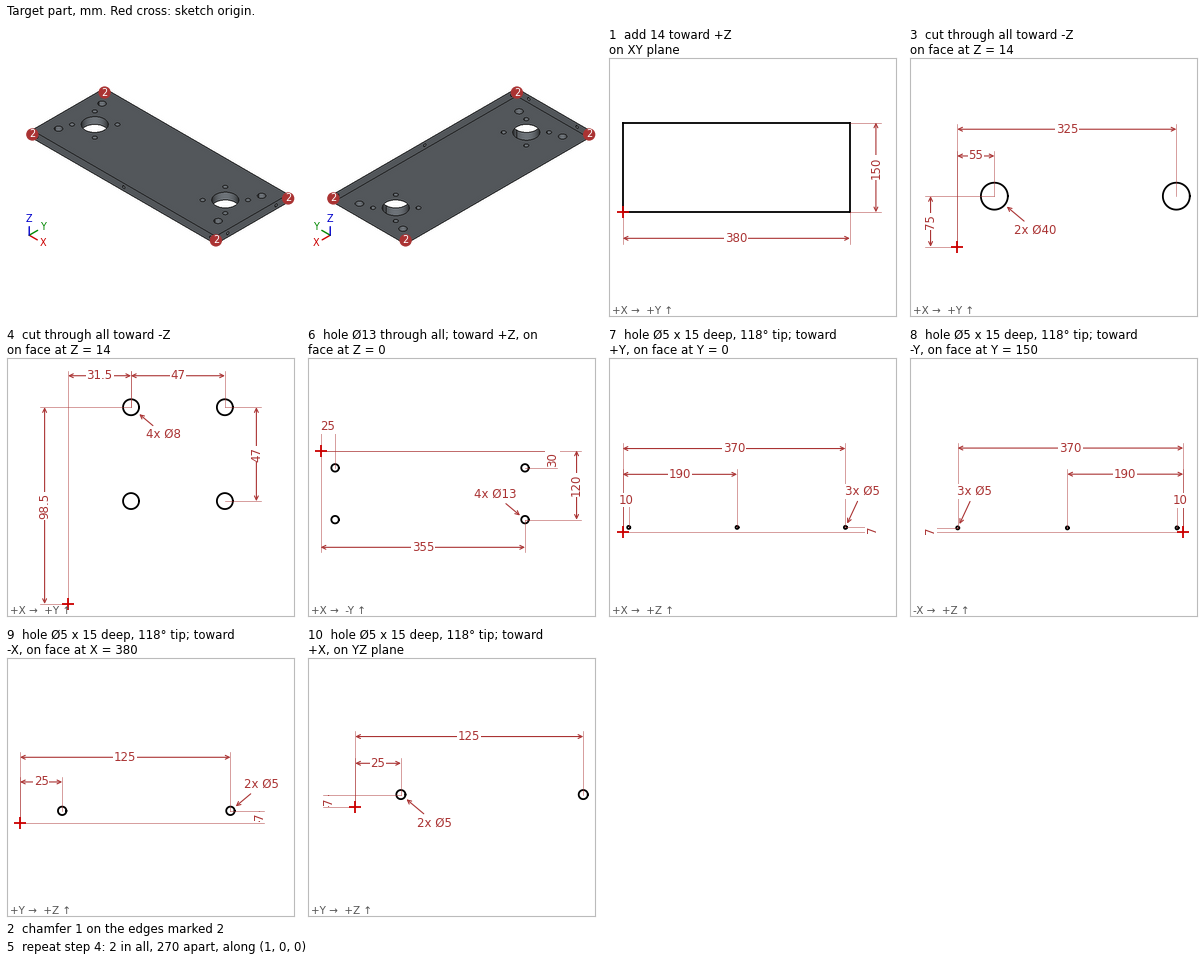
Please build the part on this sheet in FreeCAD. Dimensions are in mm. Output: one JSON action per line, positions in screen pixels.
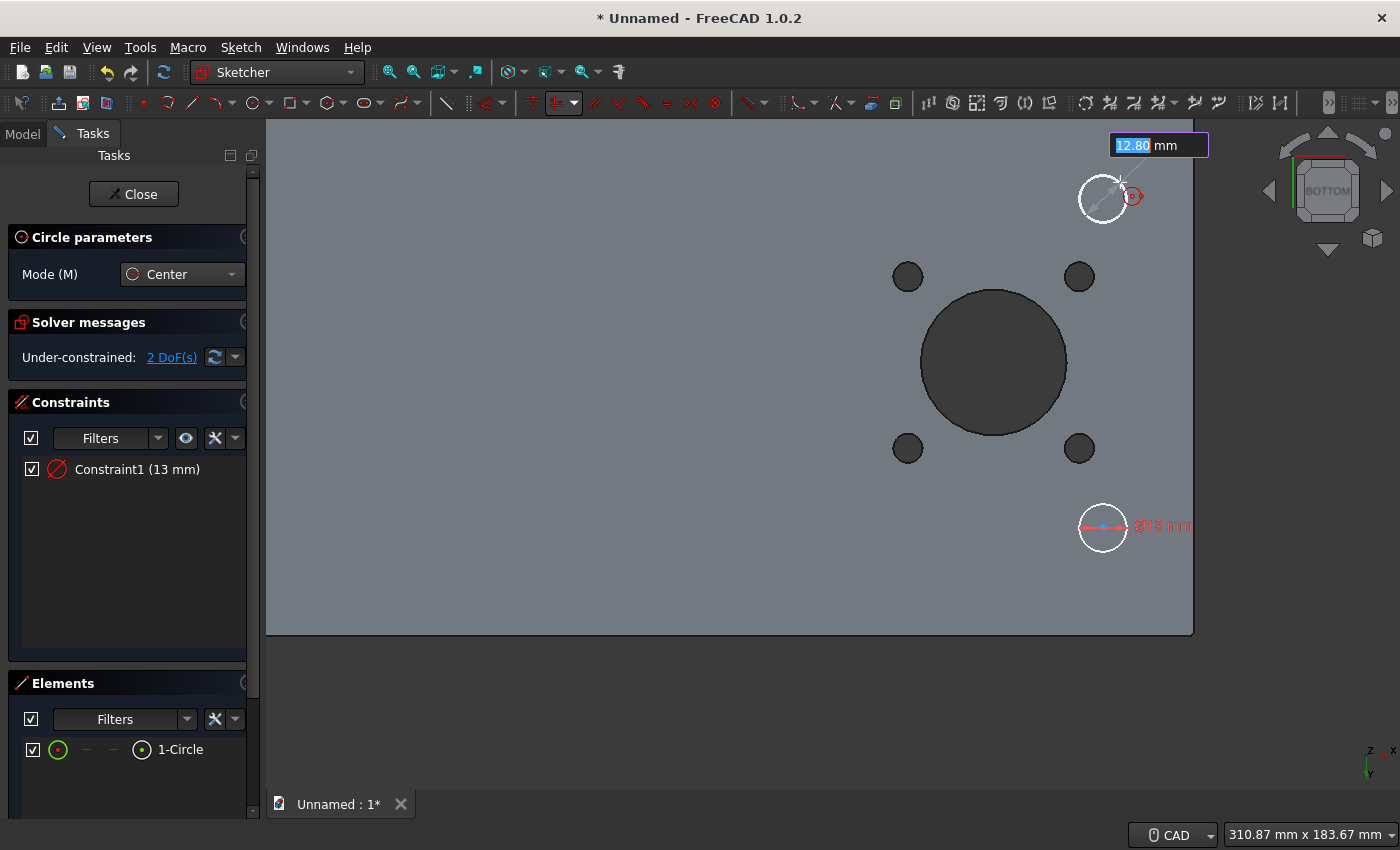
{"action": "type", "text": "13"}
{"action": "key", "text": "Return"}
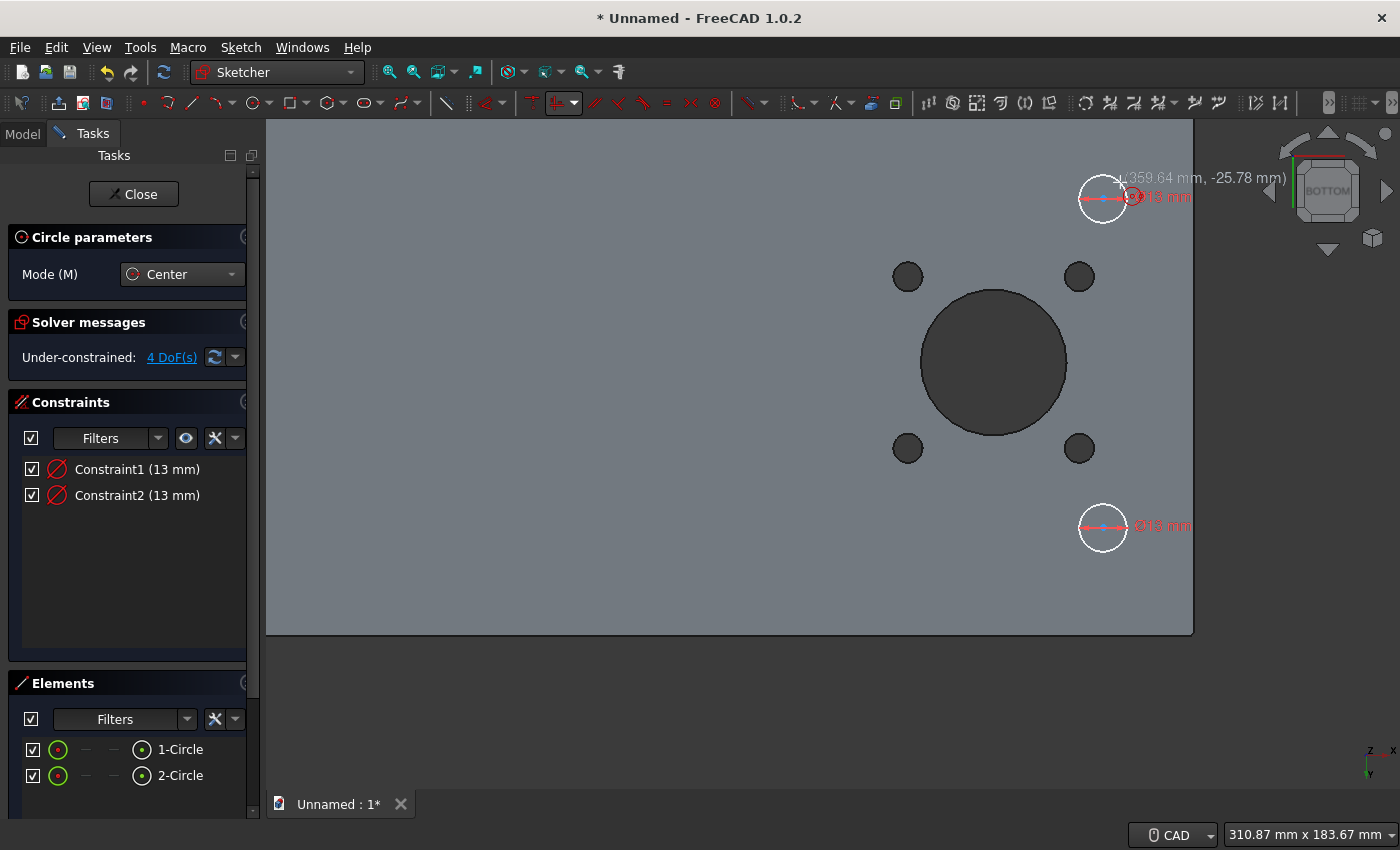
{"action": "scroll", "coordinate": [1126, 617], "scroll_direction": "down", "scroll_amount": 3}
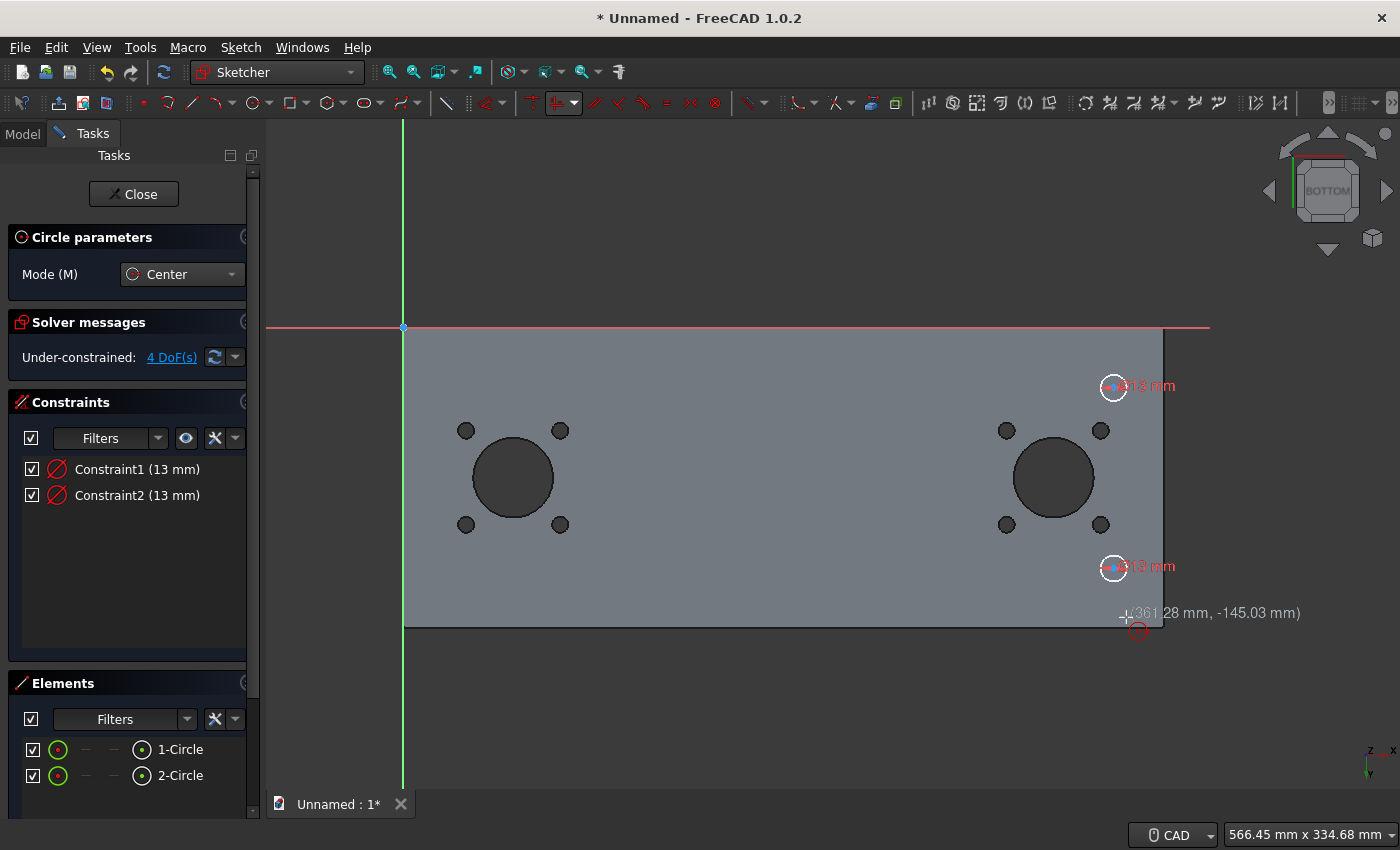
{"action": "scroll", "coordinate": [453, 388], "scroll_direction": "up", "scroll_amount": 3}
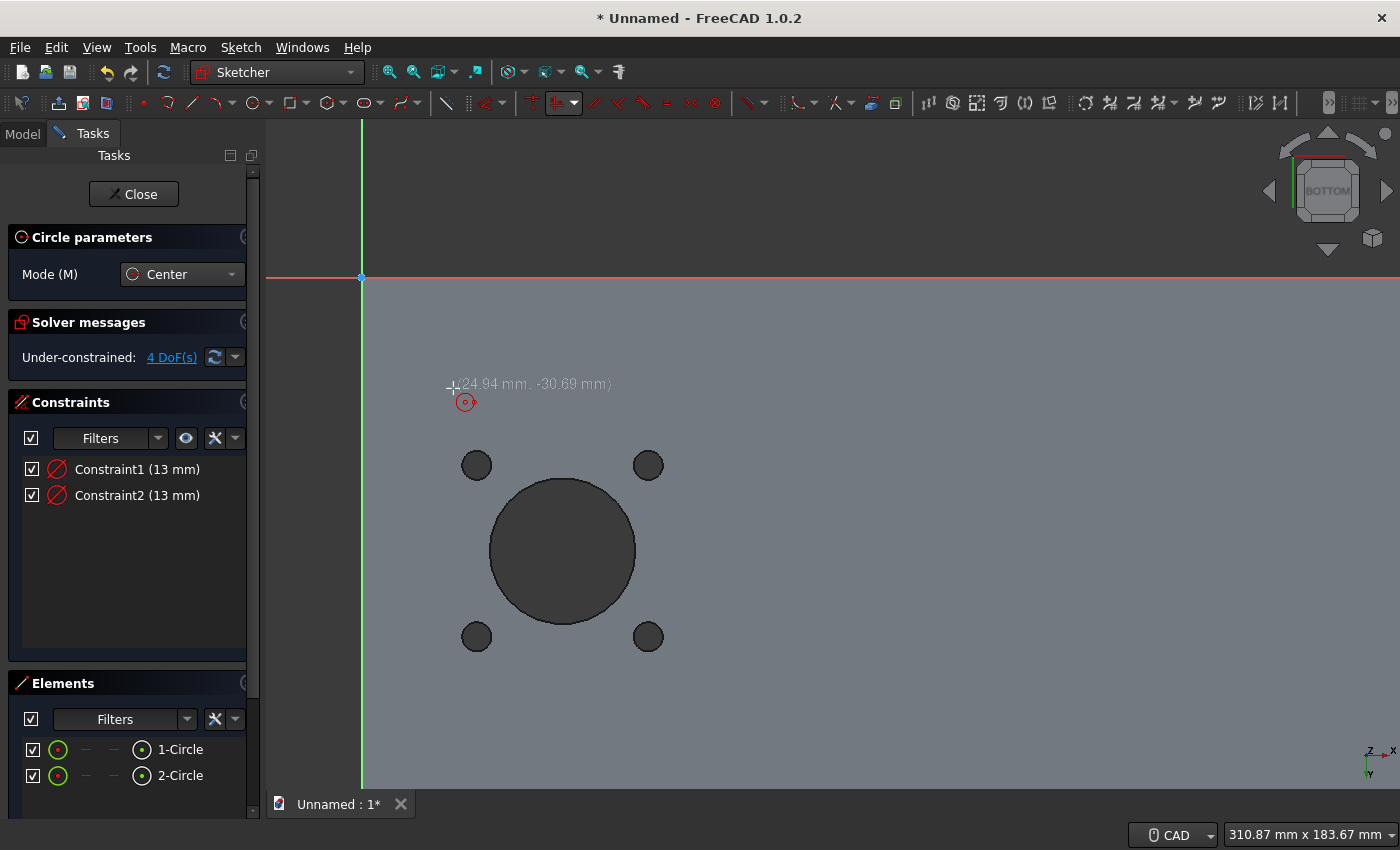
{"action": "left_click", "coordinate": [453, 387]}
{"action": "mouse_move", "coordinate": [470, 370]}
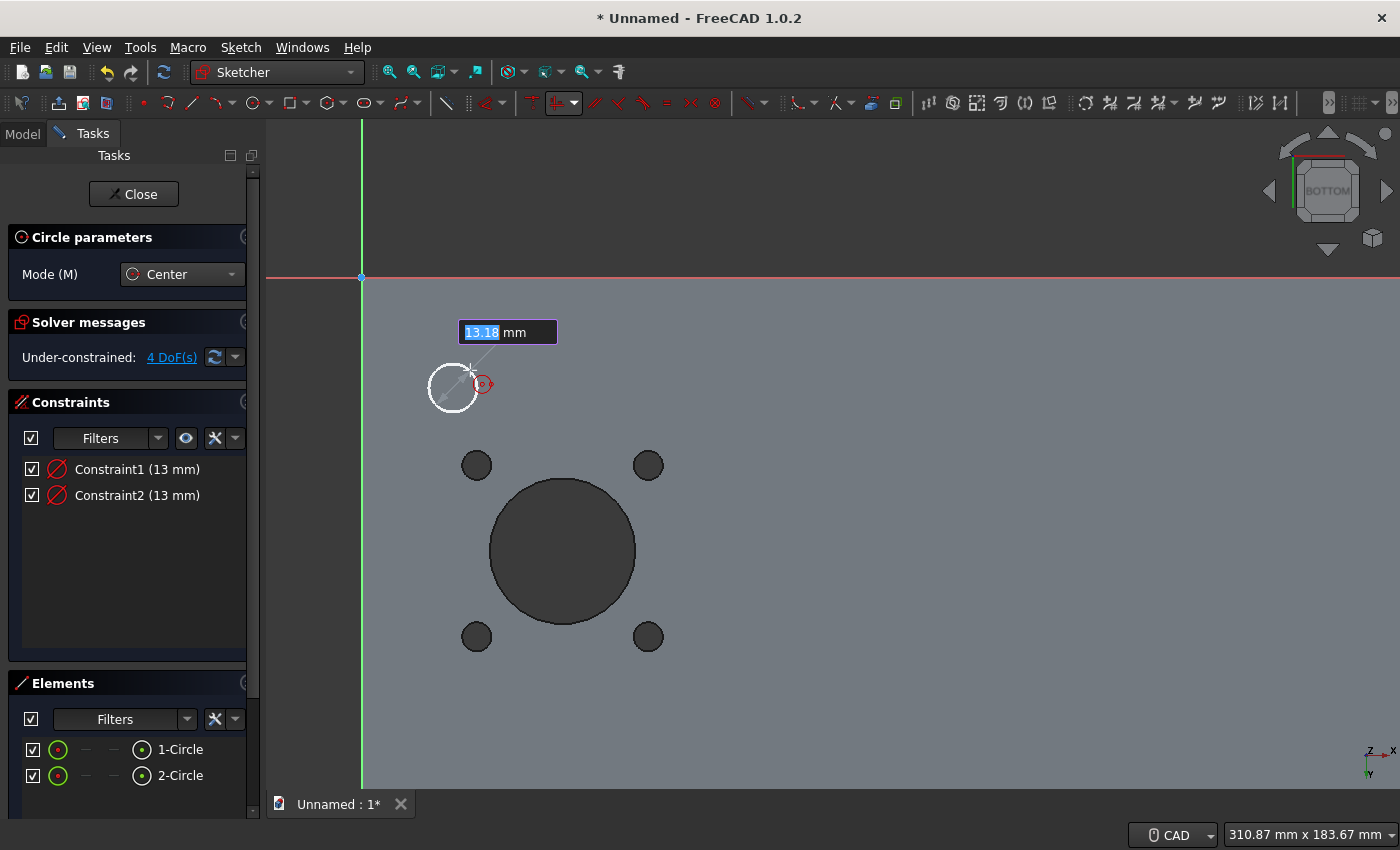
{"action": "type", "text": "13"}
{"action": "key", "text": "Return"}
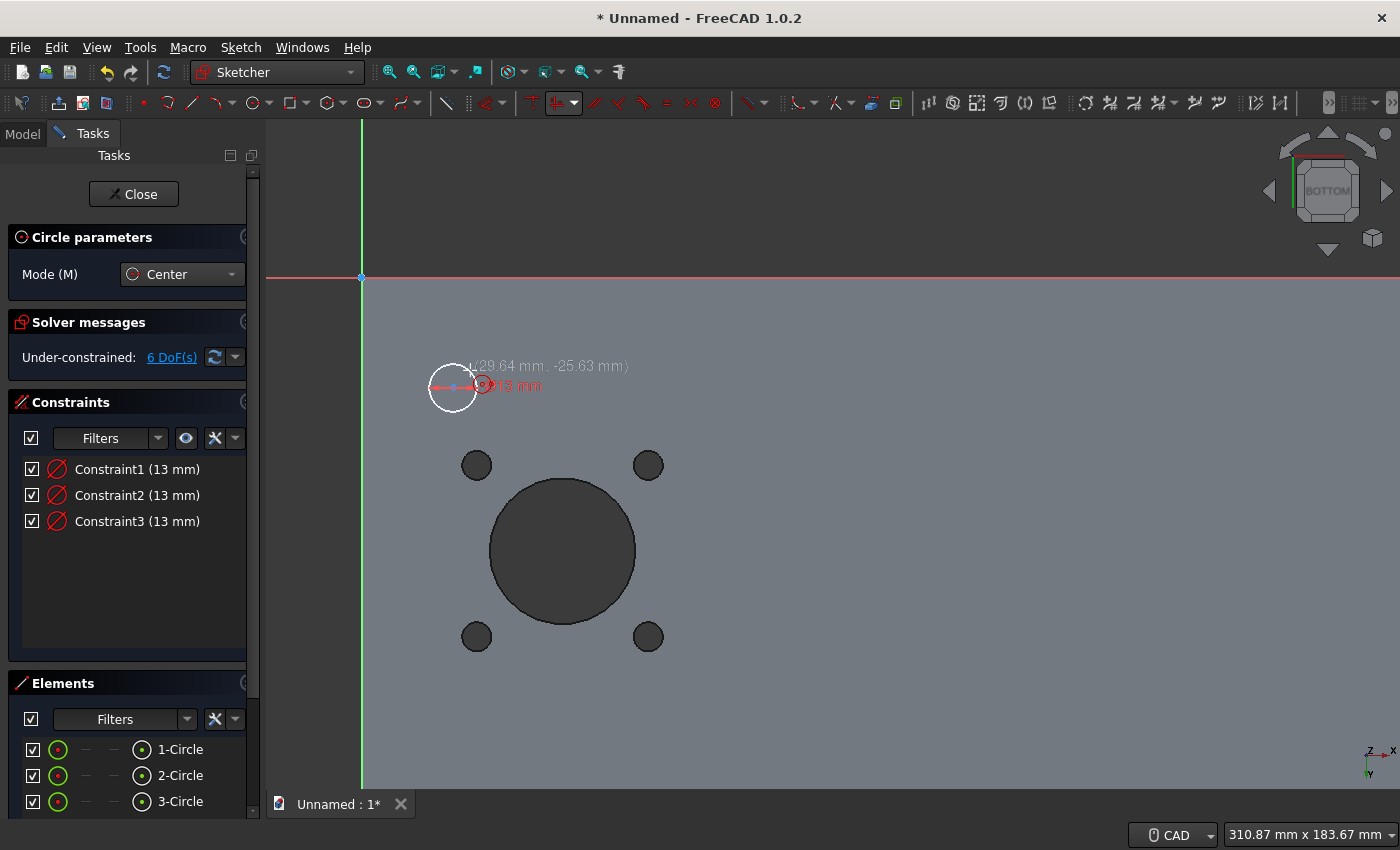
{"action": "left_click", "coordinate": [453, 715]}
{"action": "mouse_move", "coordinate": [470, 698]}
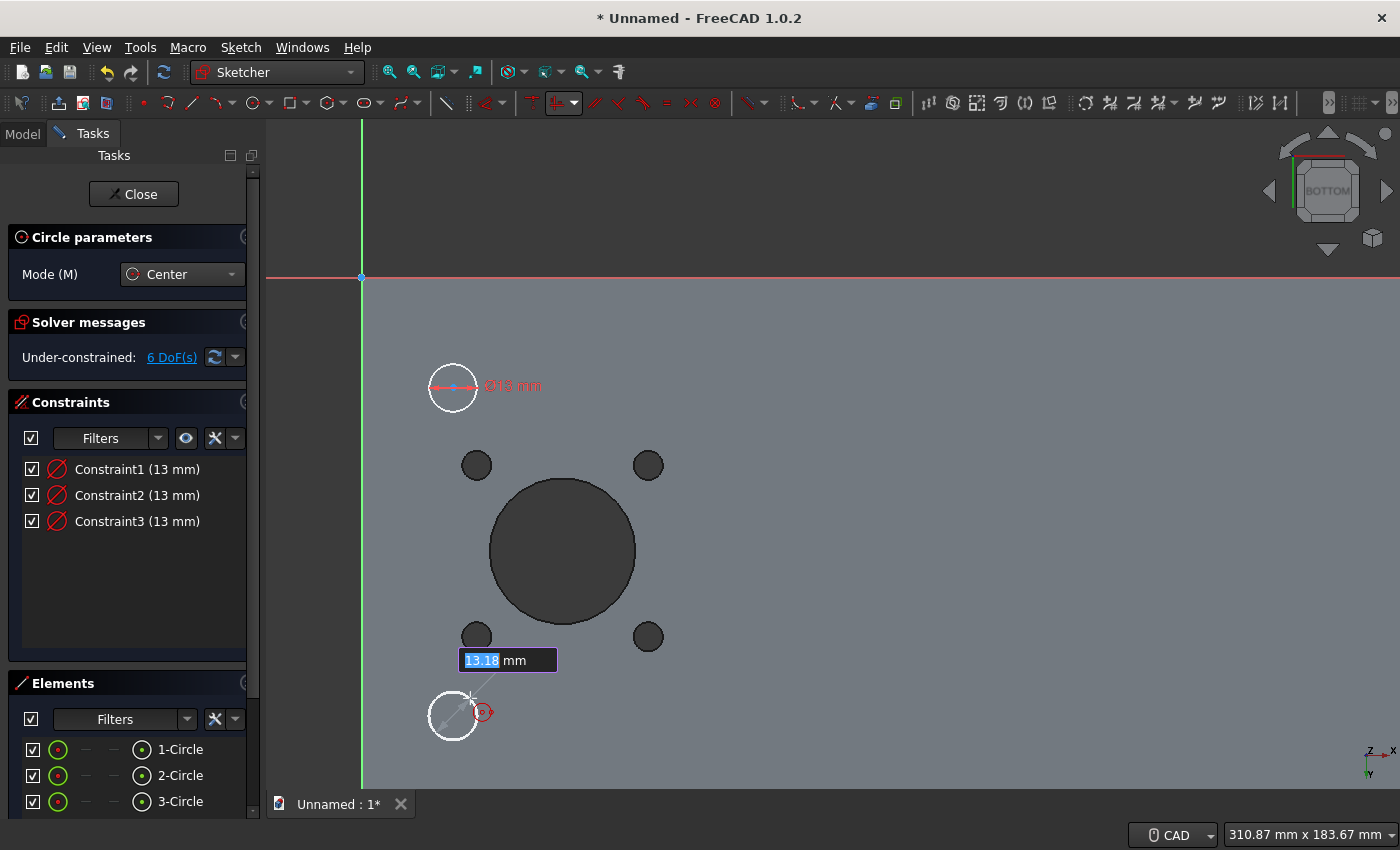
{"action": "type", "text": "13"}
{"action": "key", "text": "Return"}
{"action": "key", "text": "Escape"}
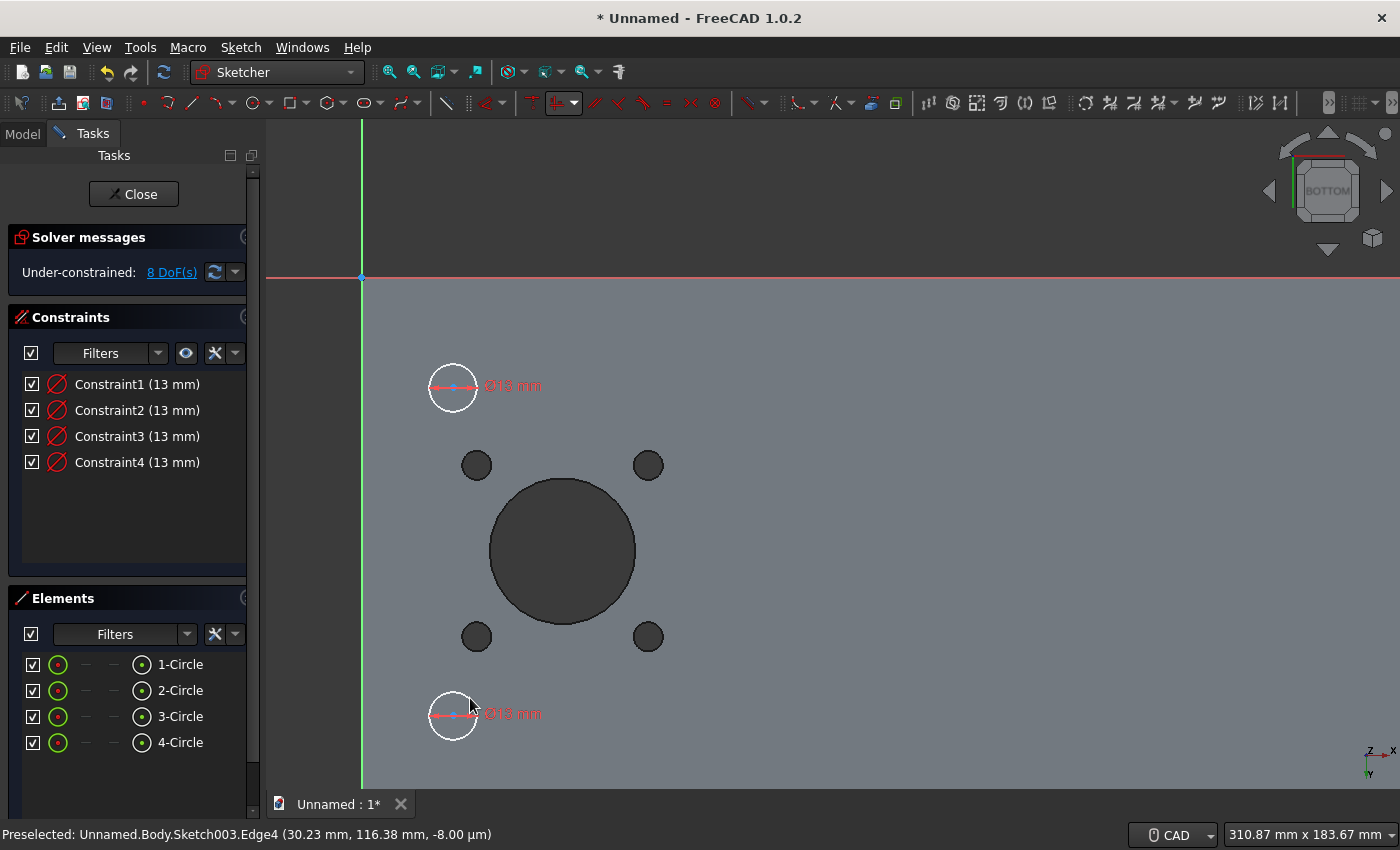
{"action": "scroll", "coordinate": [452, 388], "scroll_direction": "down", "scroll_amount": 3}